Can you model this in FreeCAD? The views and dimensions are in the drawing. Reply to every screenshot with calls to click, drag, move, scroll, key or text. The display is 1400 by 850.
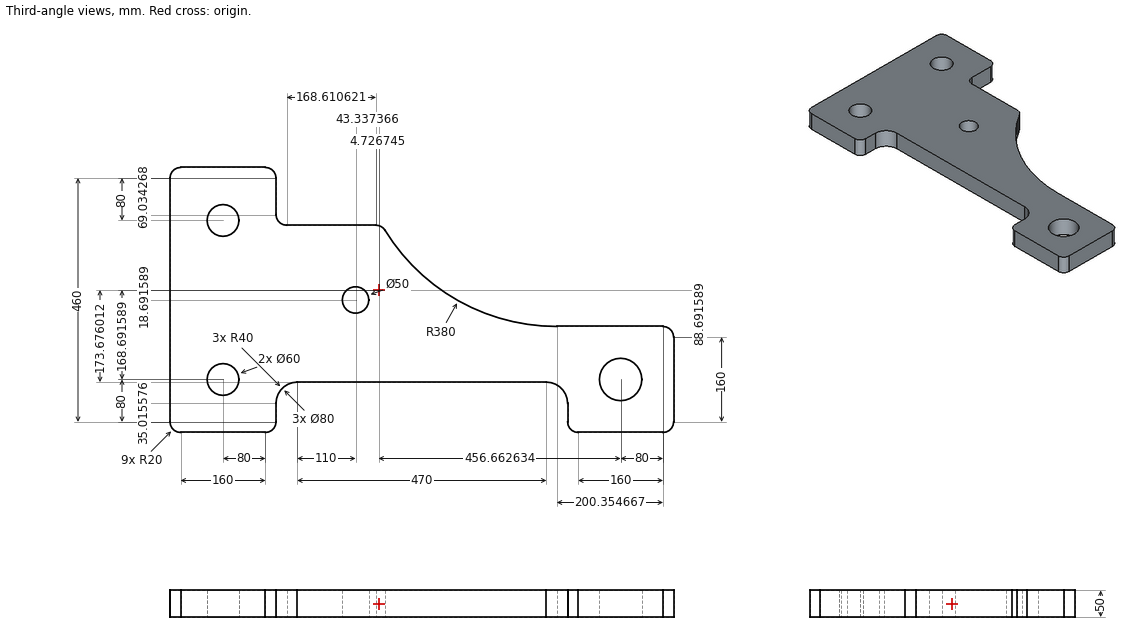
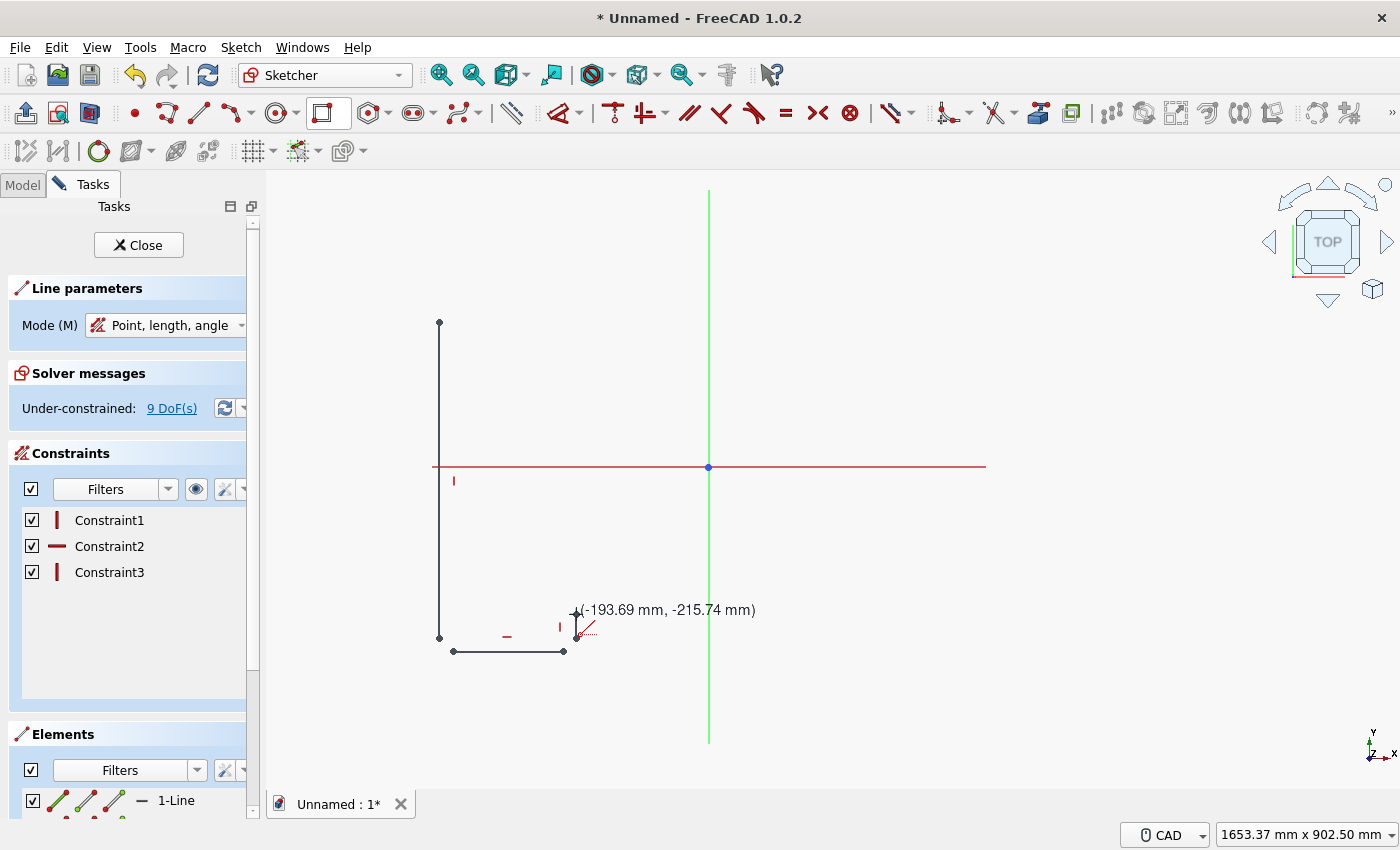
click(604, 586)
click(926, 586)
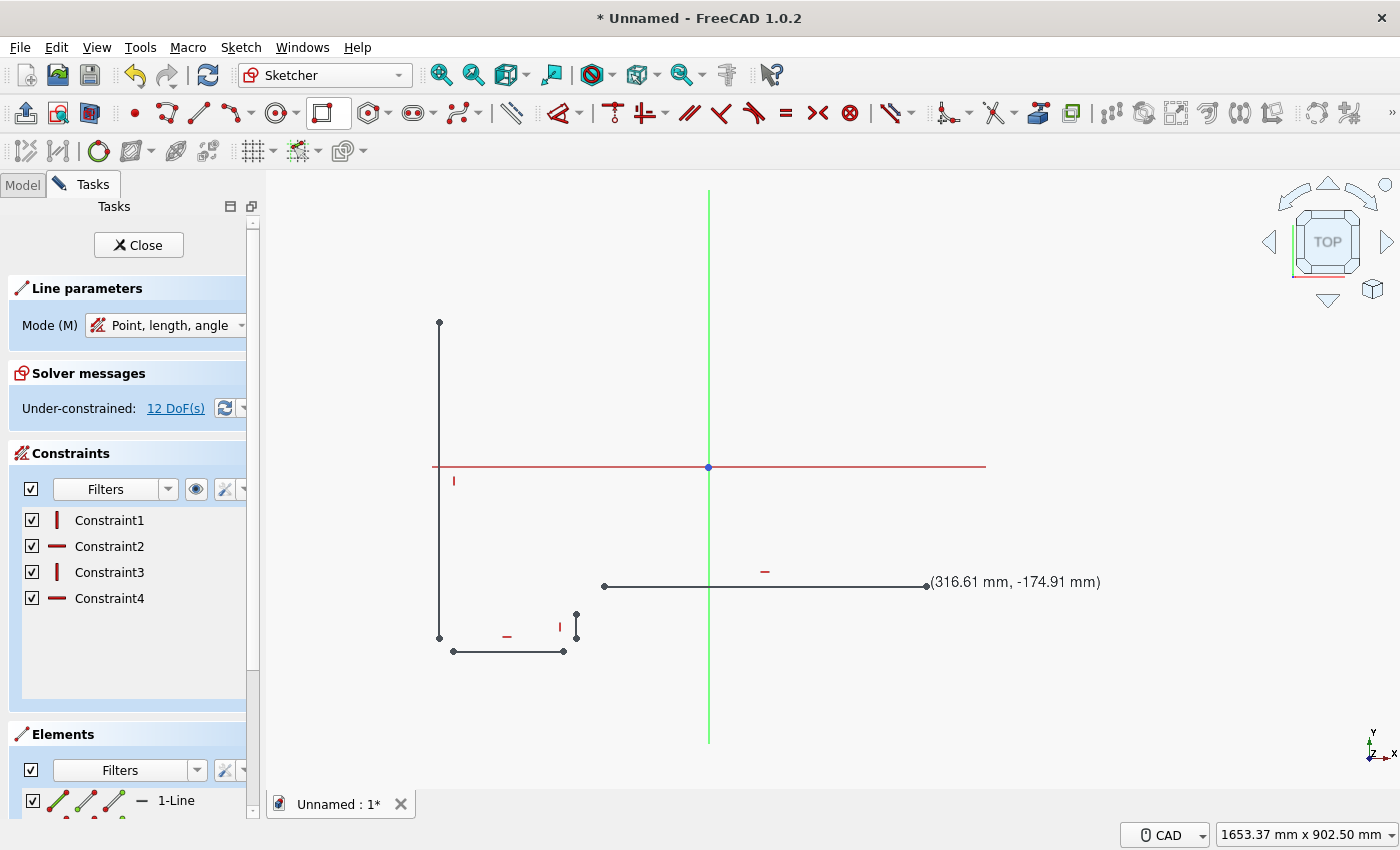
click(953, 614)
click(953, 638)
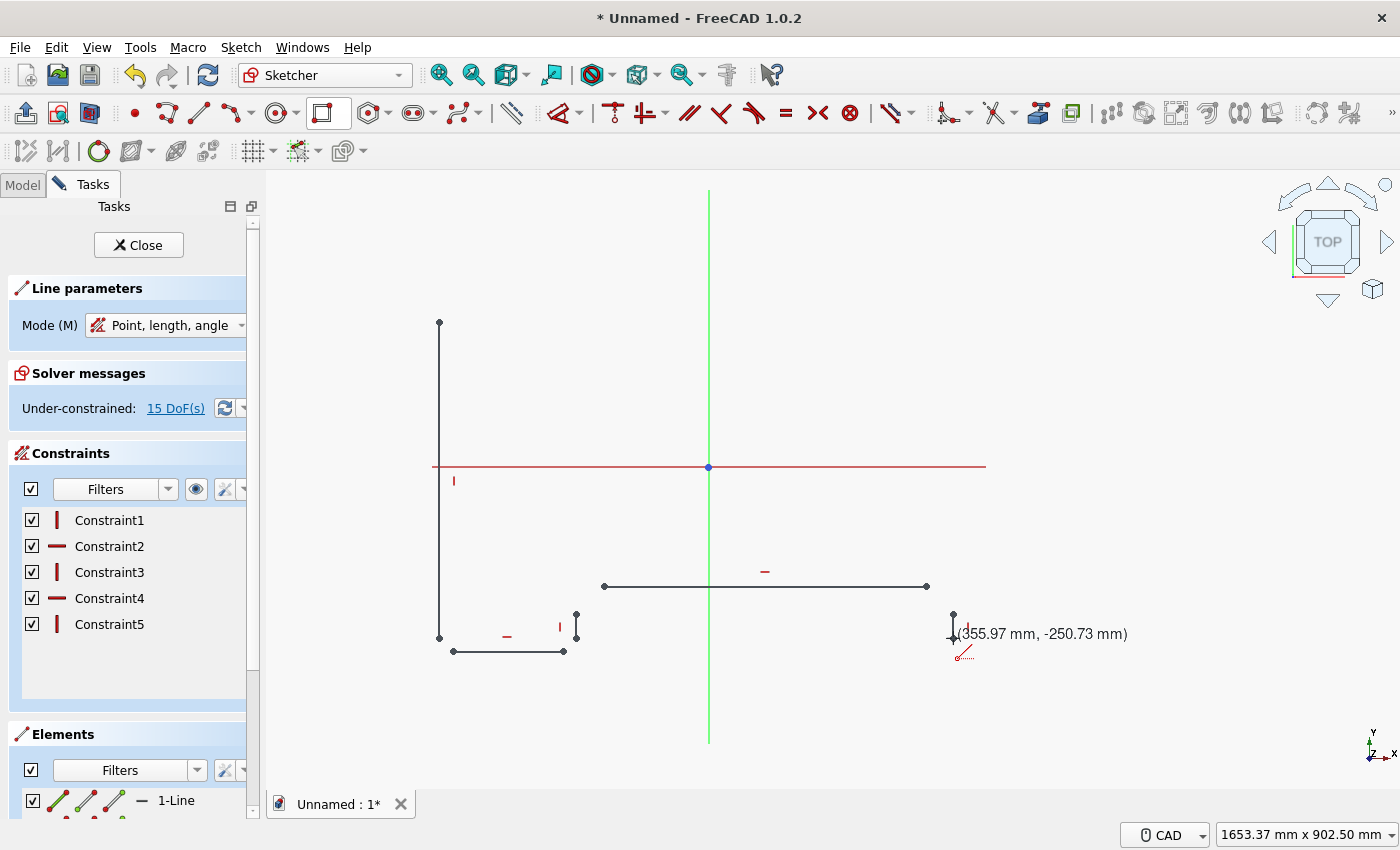
click(967, 651)
click(1077, 651)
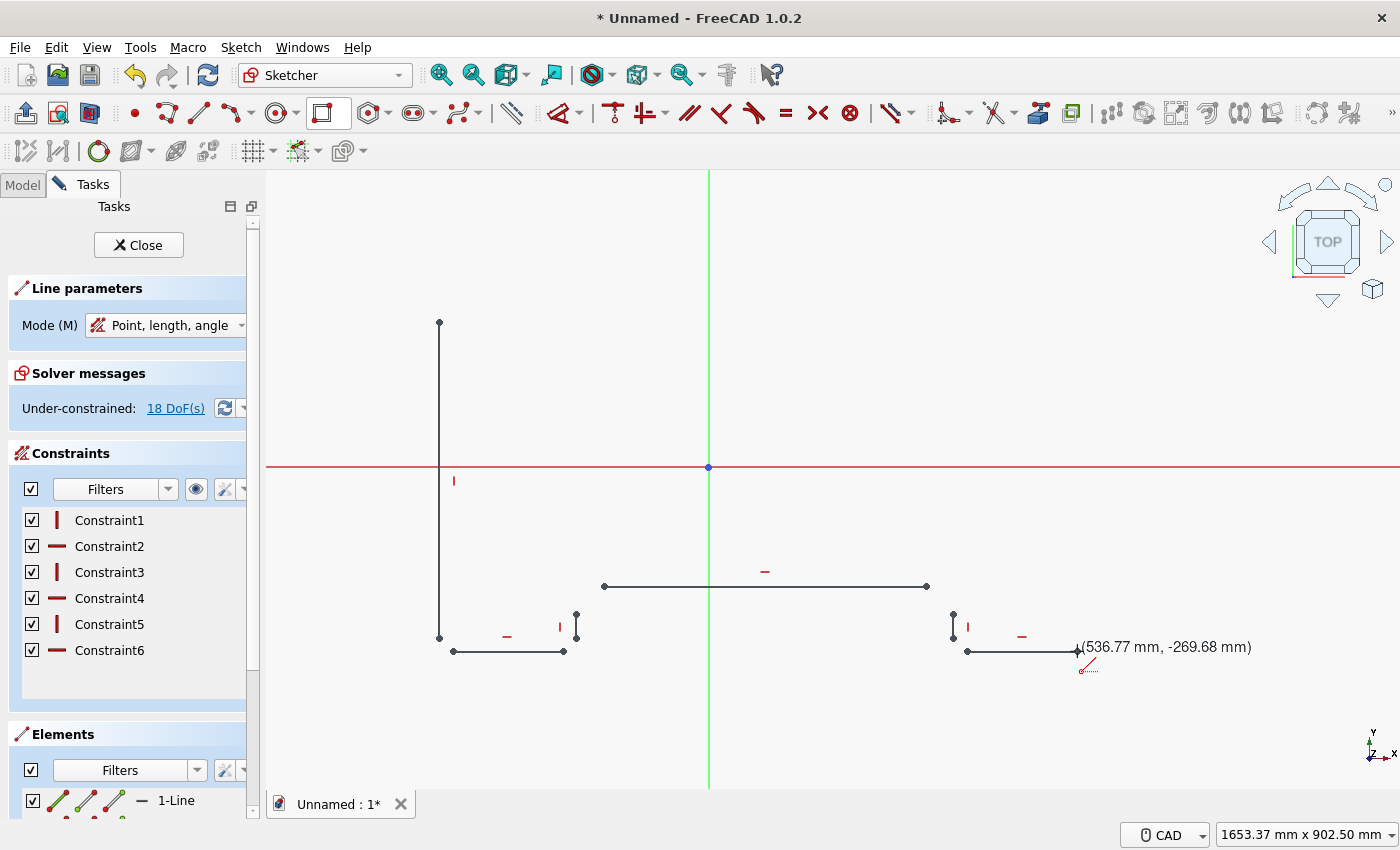
click(1091, 638)
click(1091, 528)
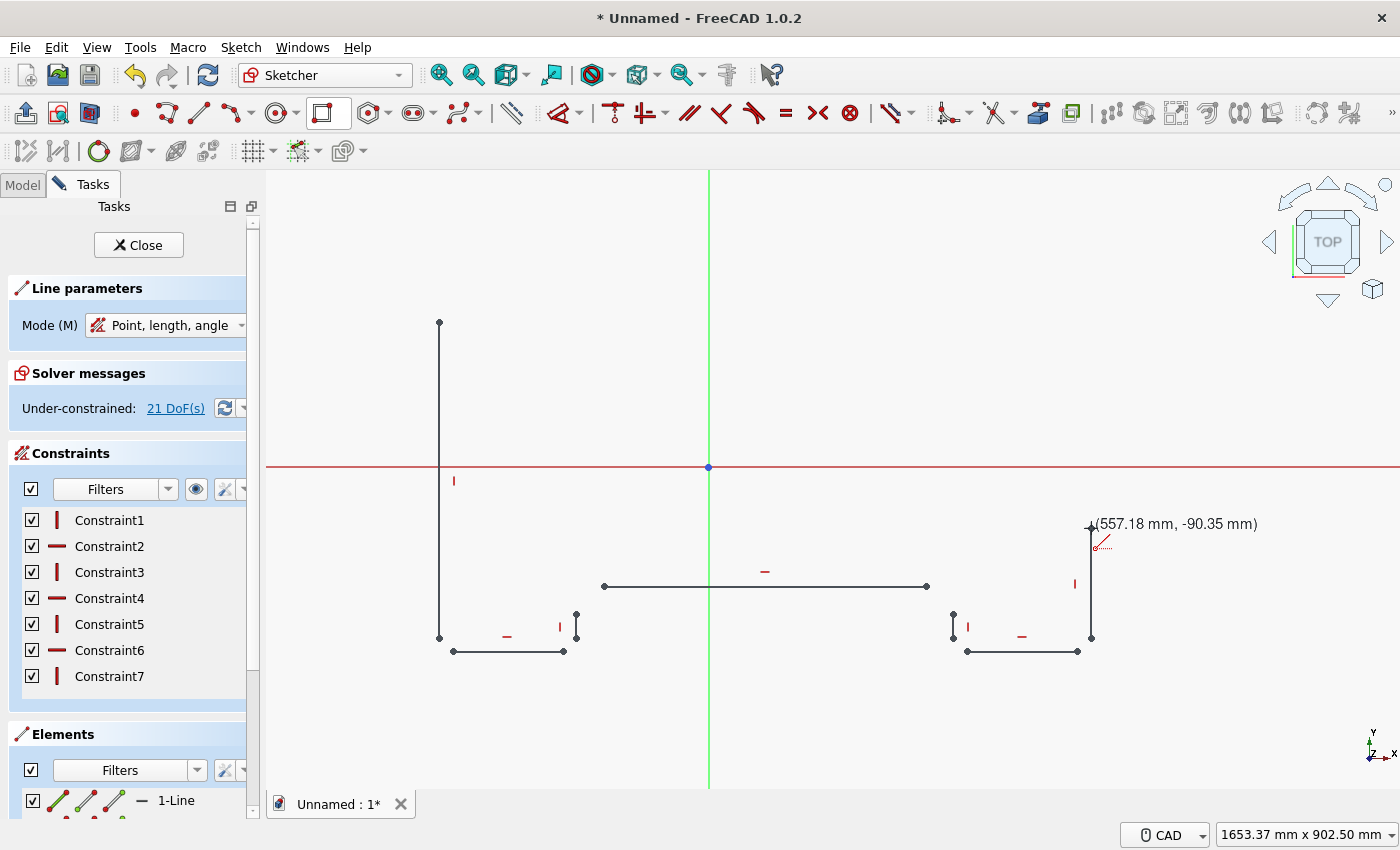
click(1077, 514)
click(940, 514)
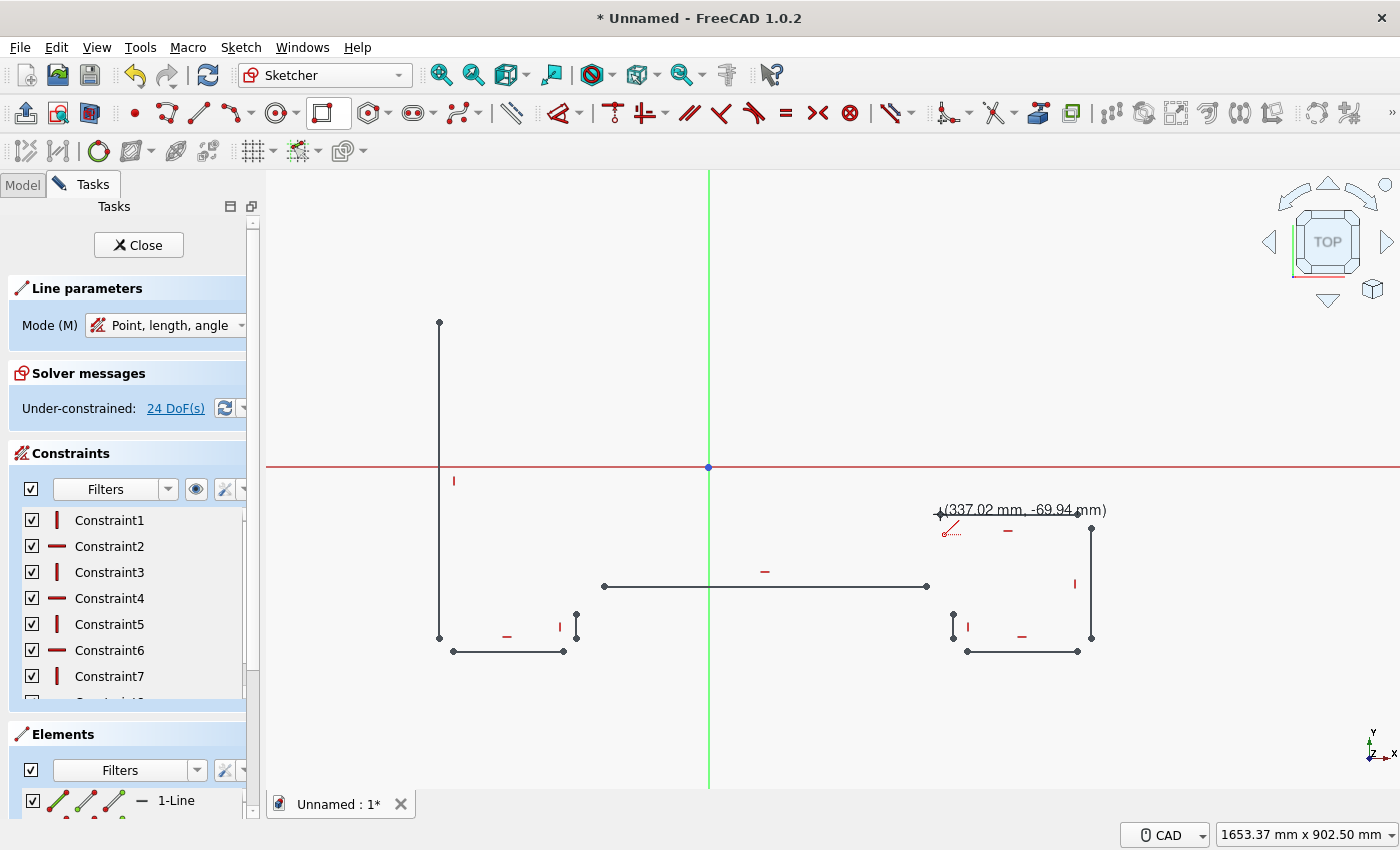
scroll(706, 383, up, 8)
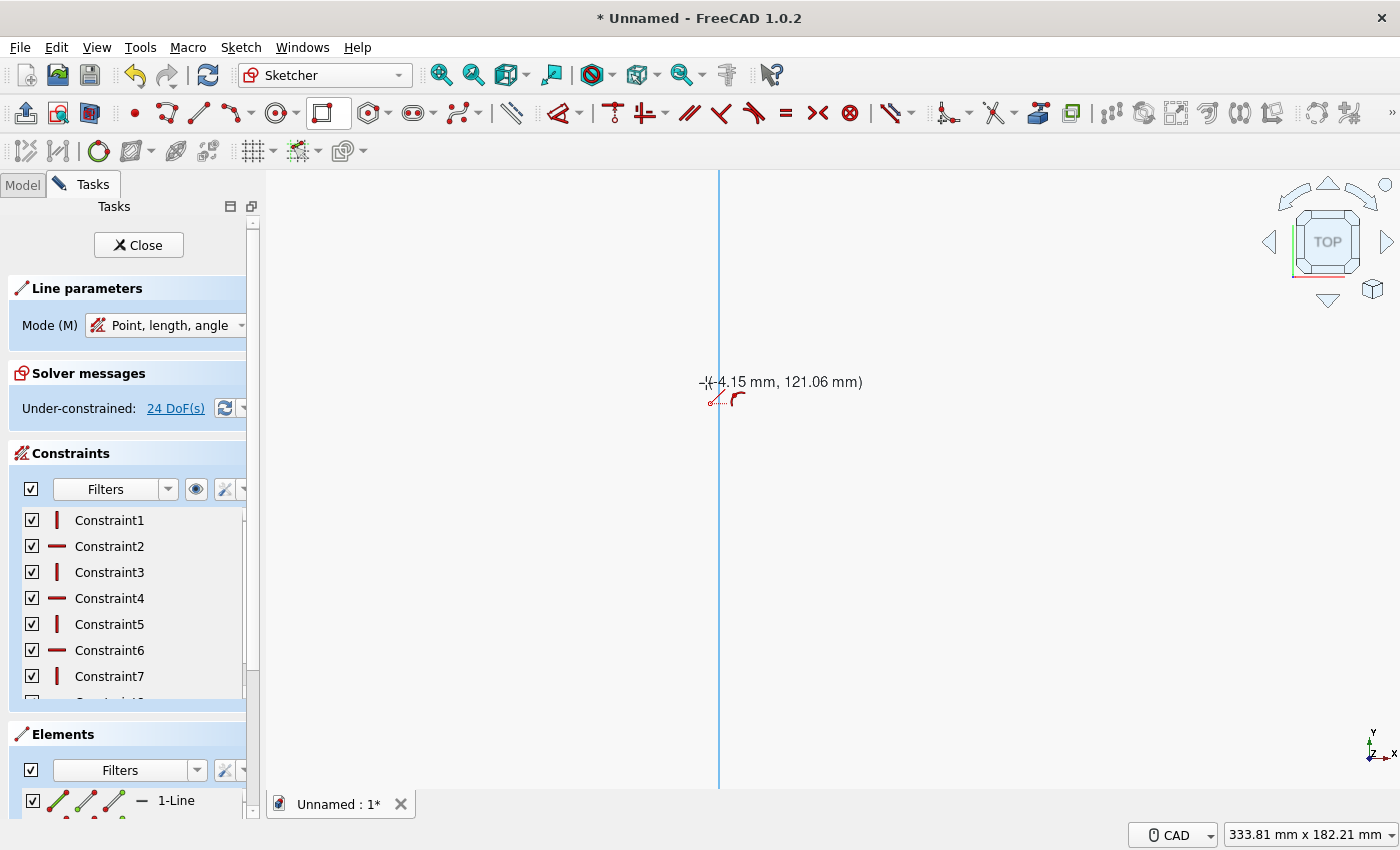
click(703, 382)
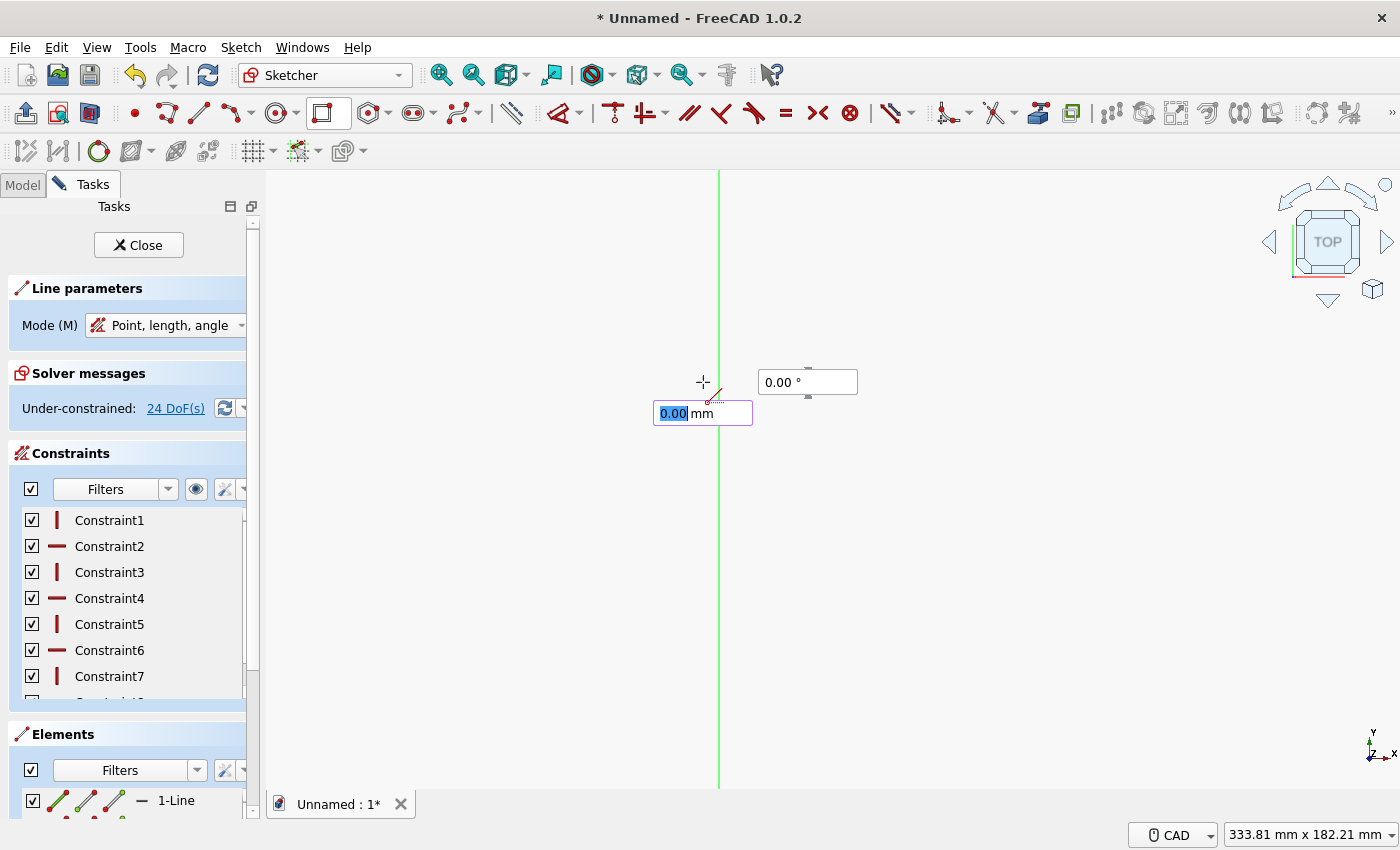
scroll(706, 383, down, 8)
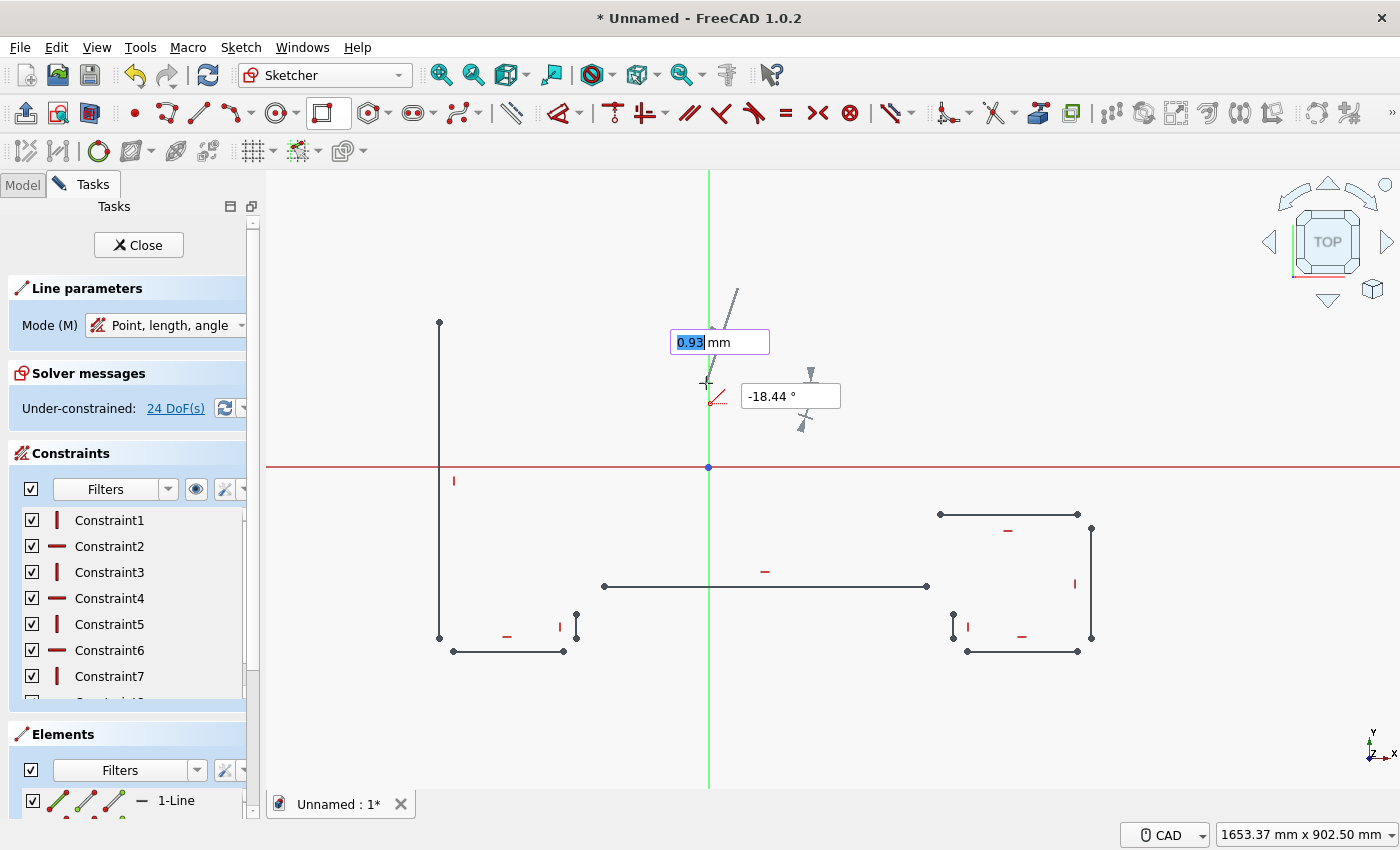
click(590, 383)